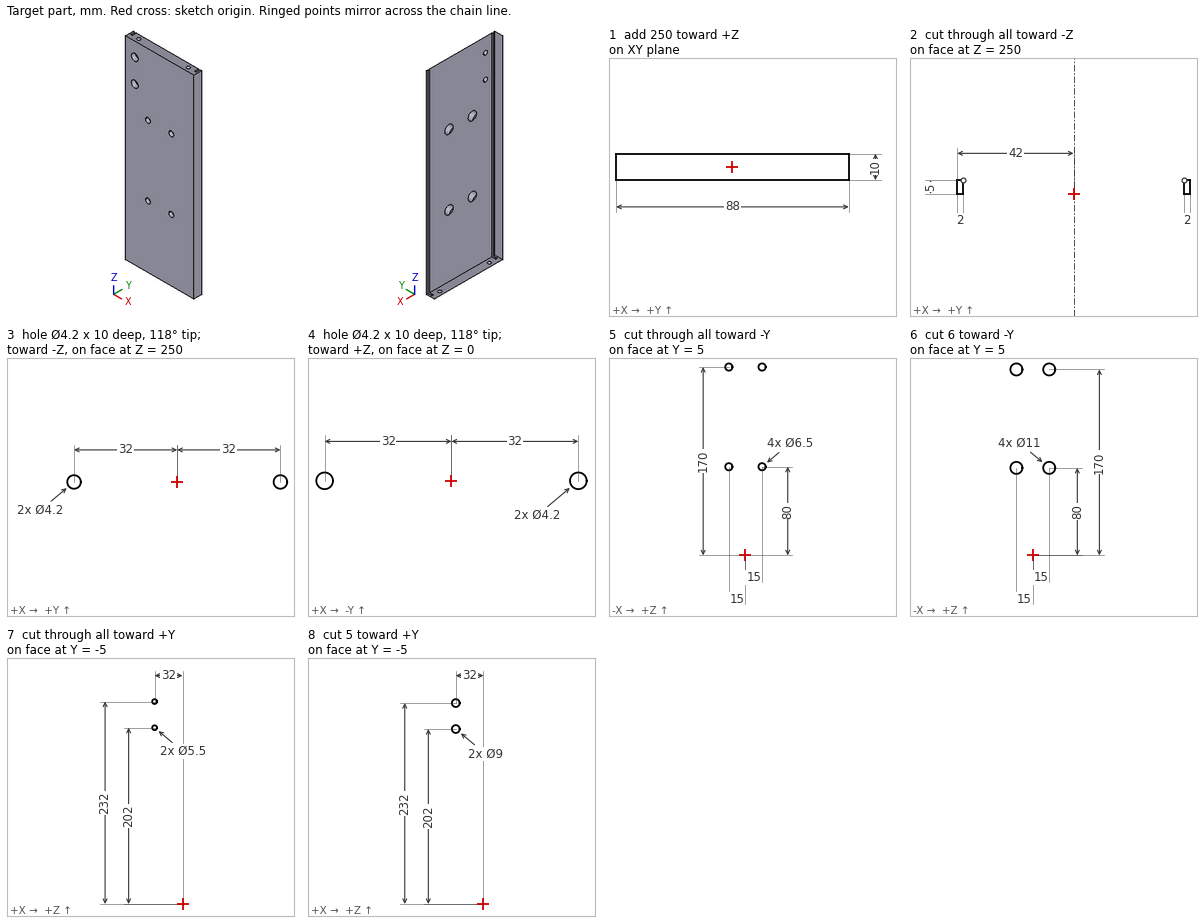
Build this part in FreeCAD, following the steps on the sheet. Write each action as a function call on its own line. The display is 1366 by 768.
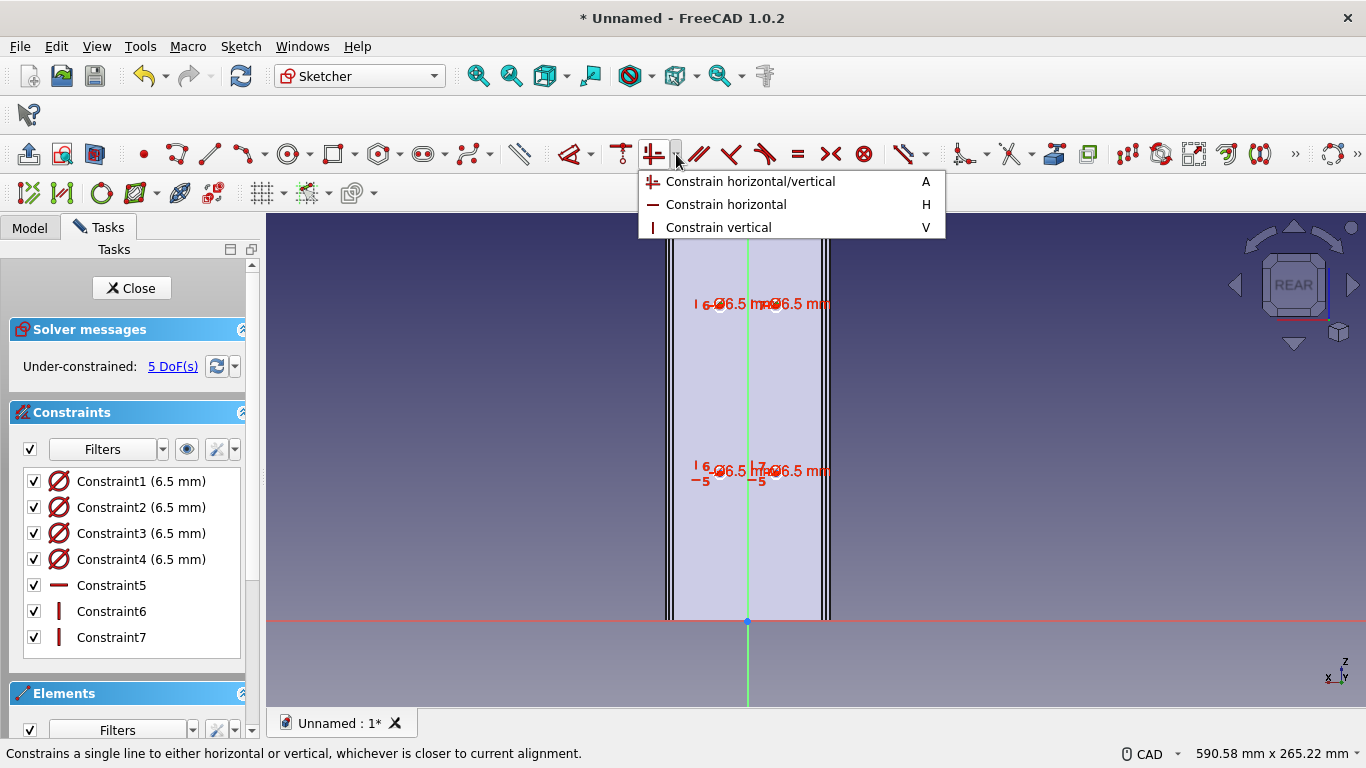
click(792, 204)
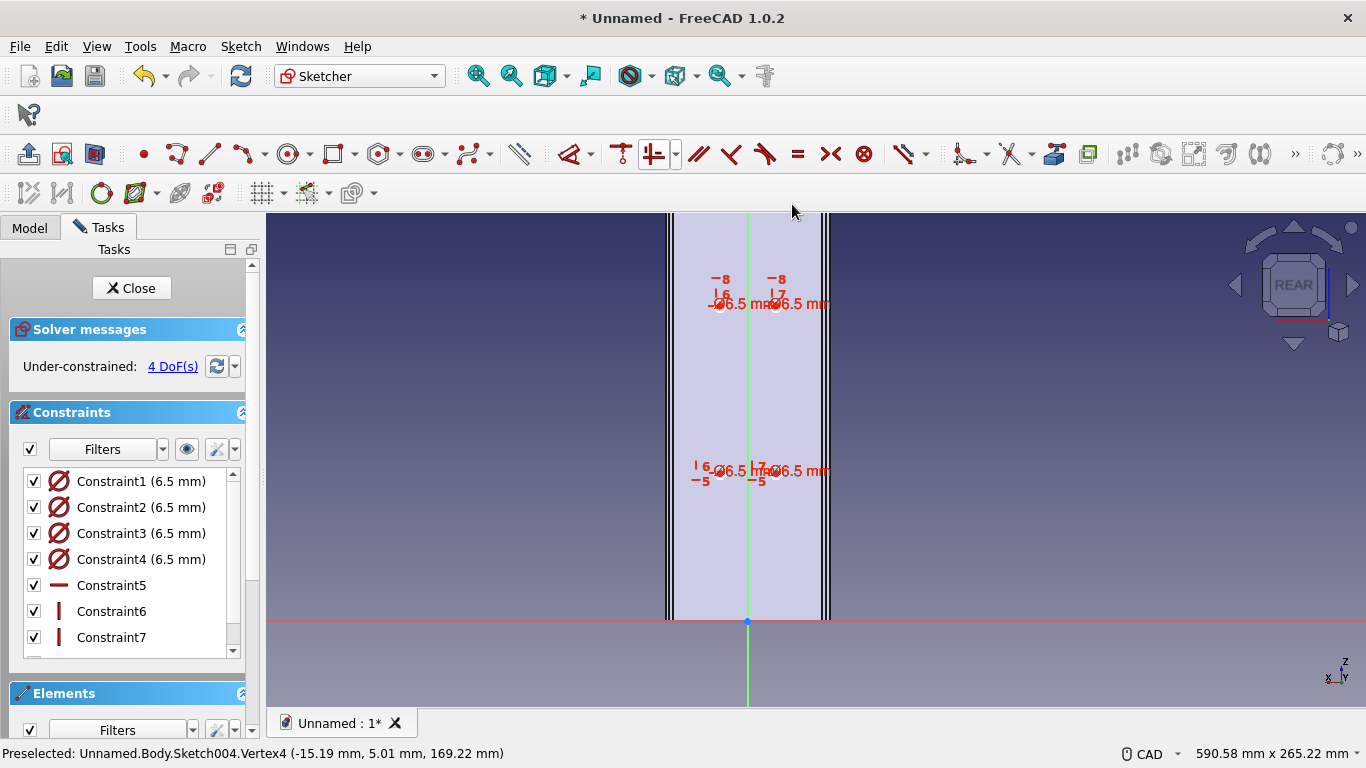
click(568, 154)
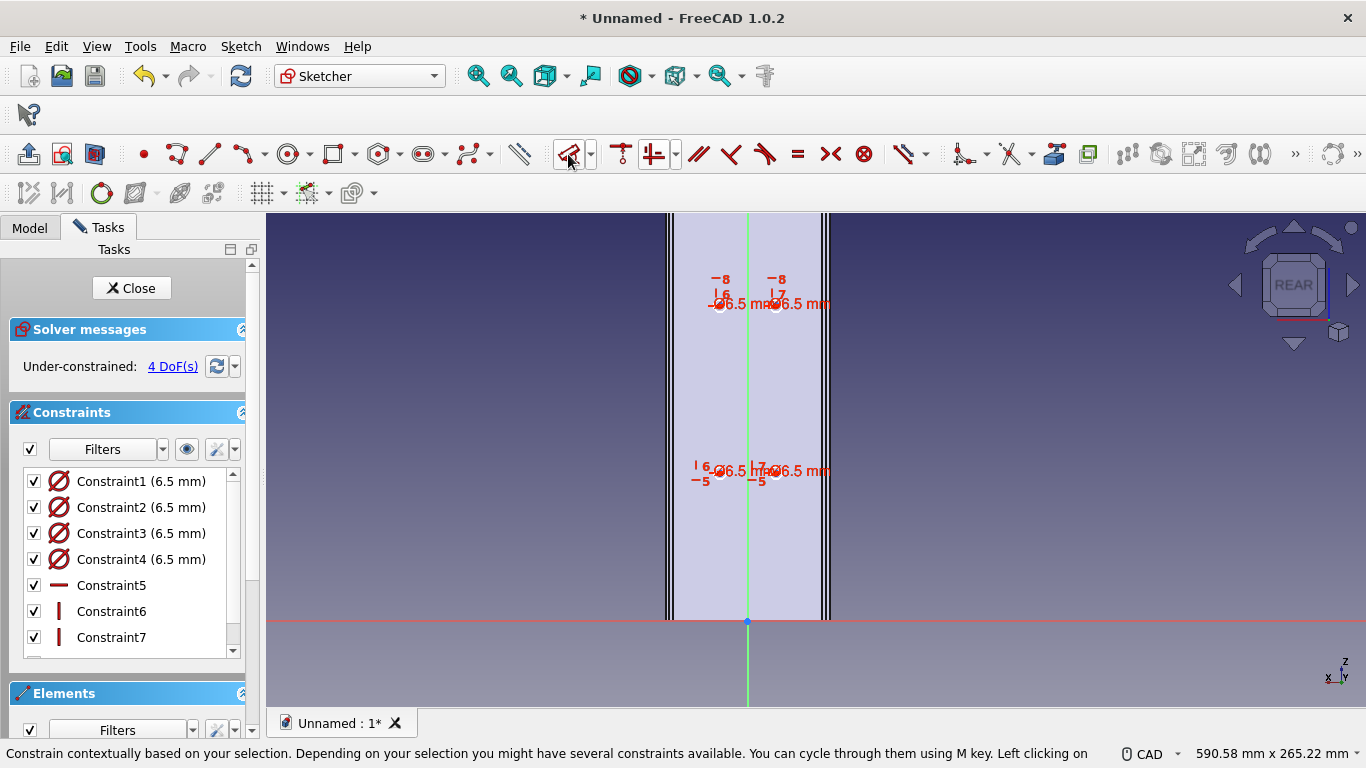
scroll(776, 473, up, 2)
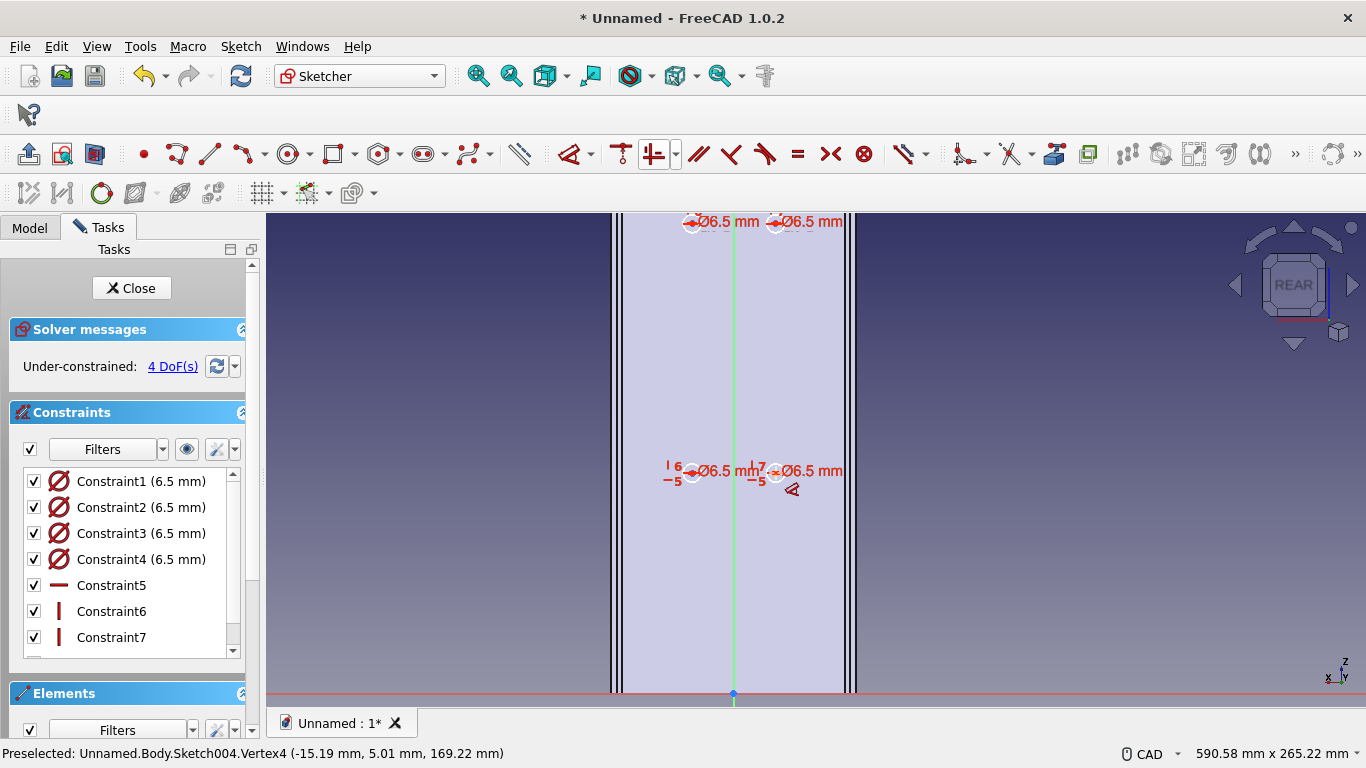
click(776, 473)
click(755, 439)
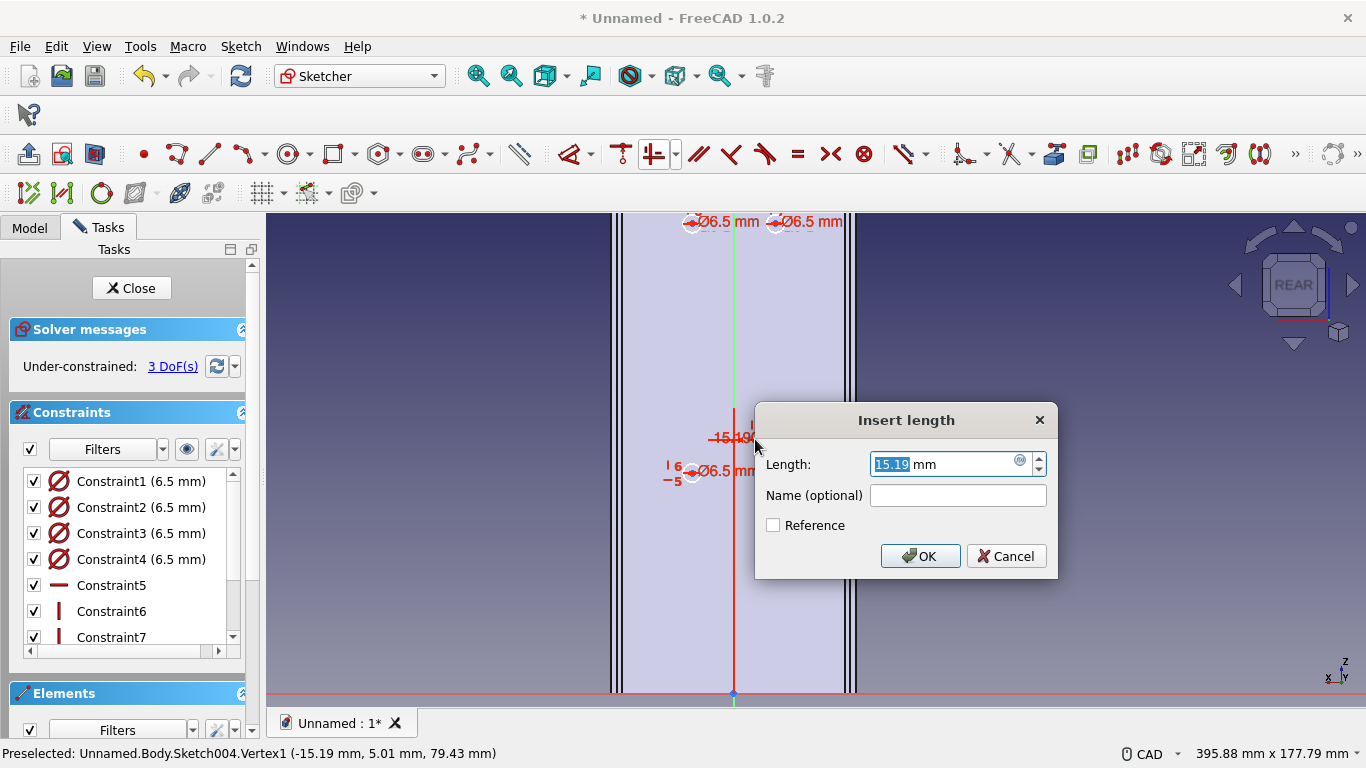
text(15)
key(Return)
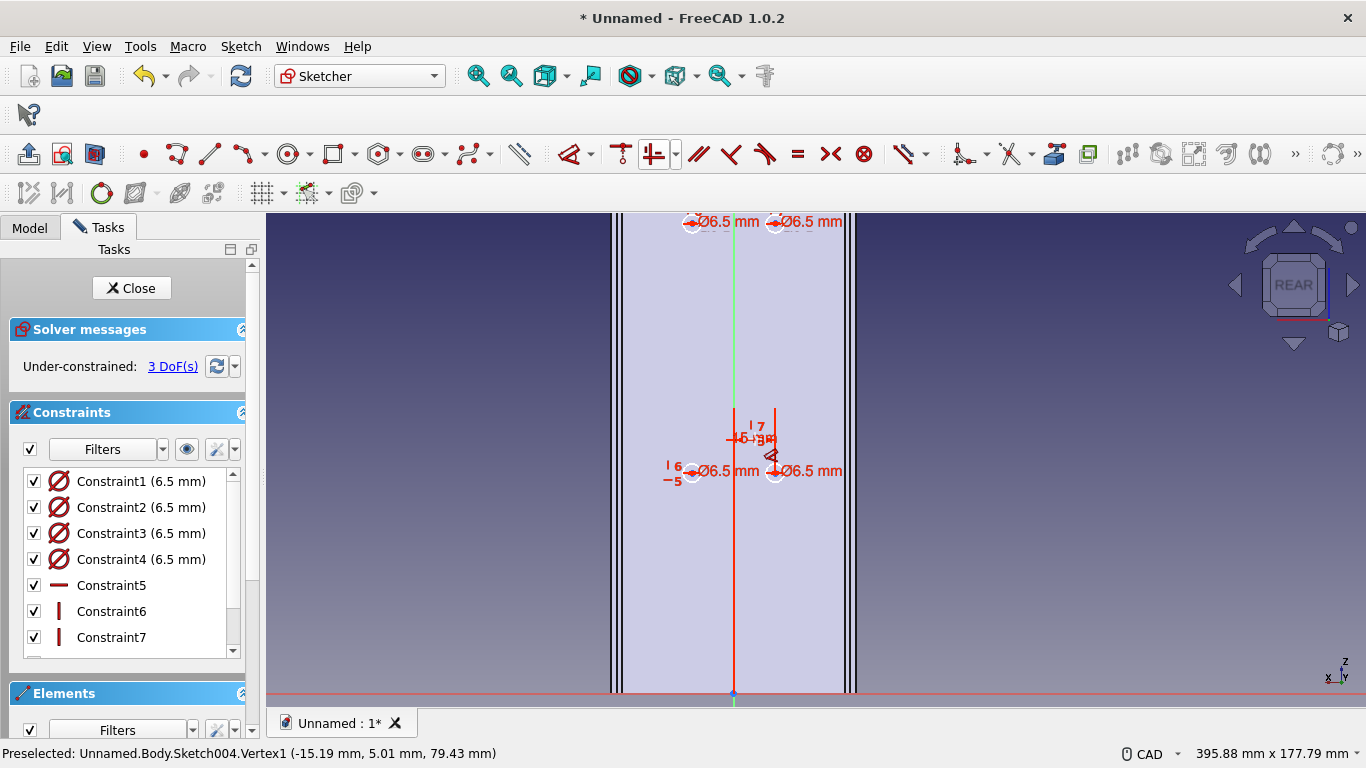
click(775, 473)
click(809, 576)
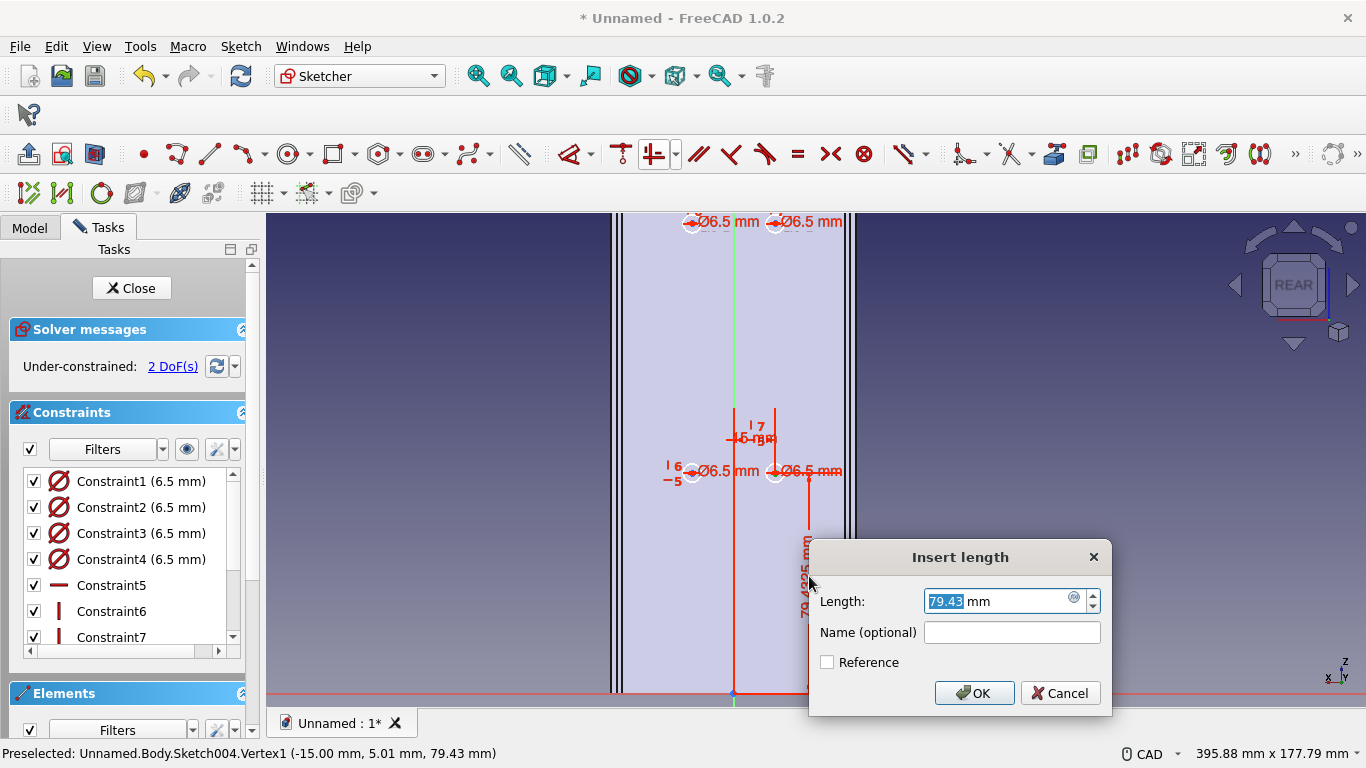
text(80)
key(Return)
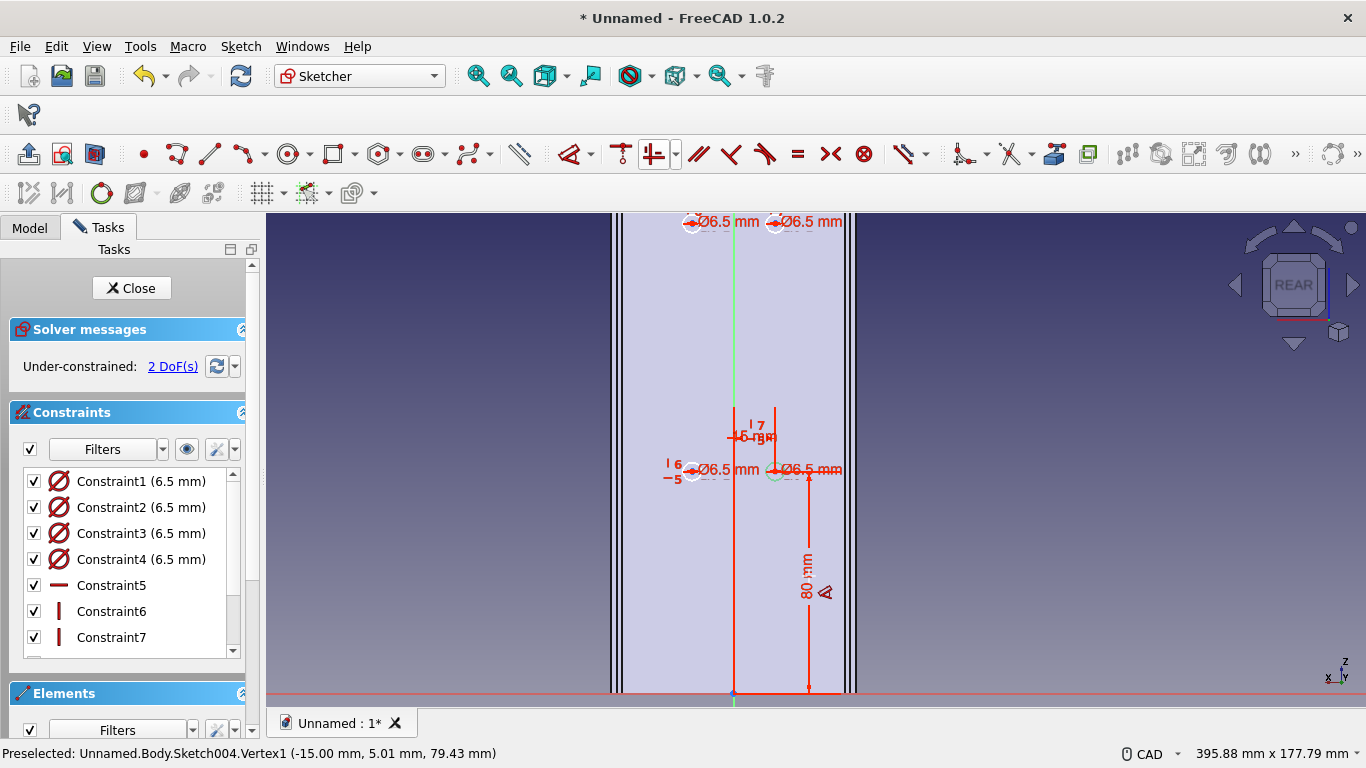
click(692, 472)
click(713, 414)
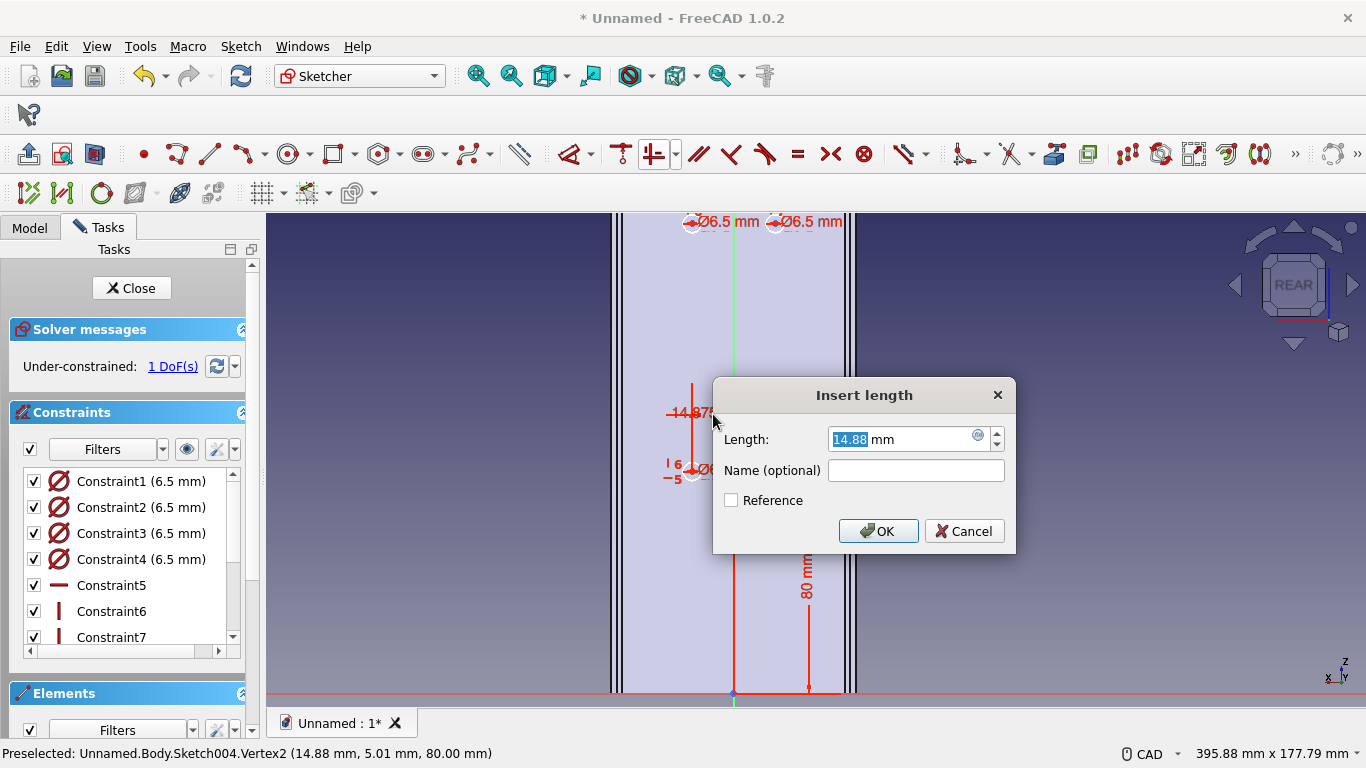
text(15)
key(Return)